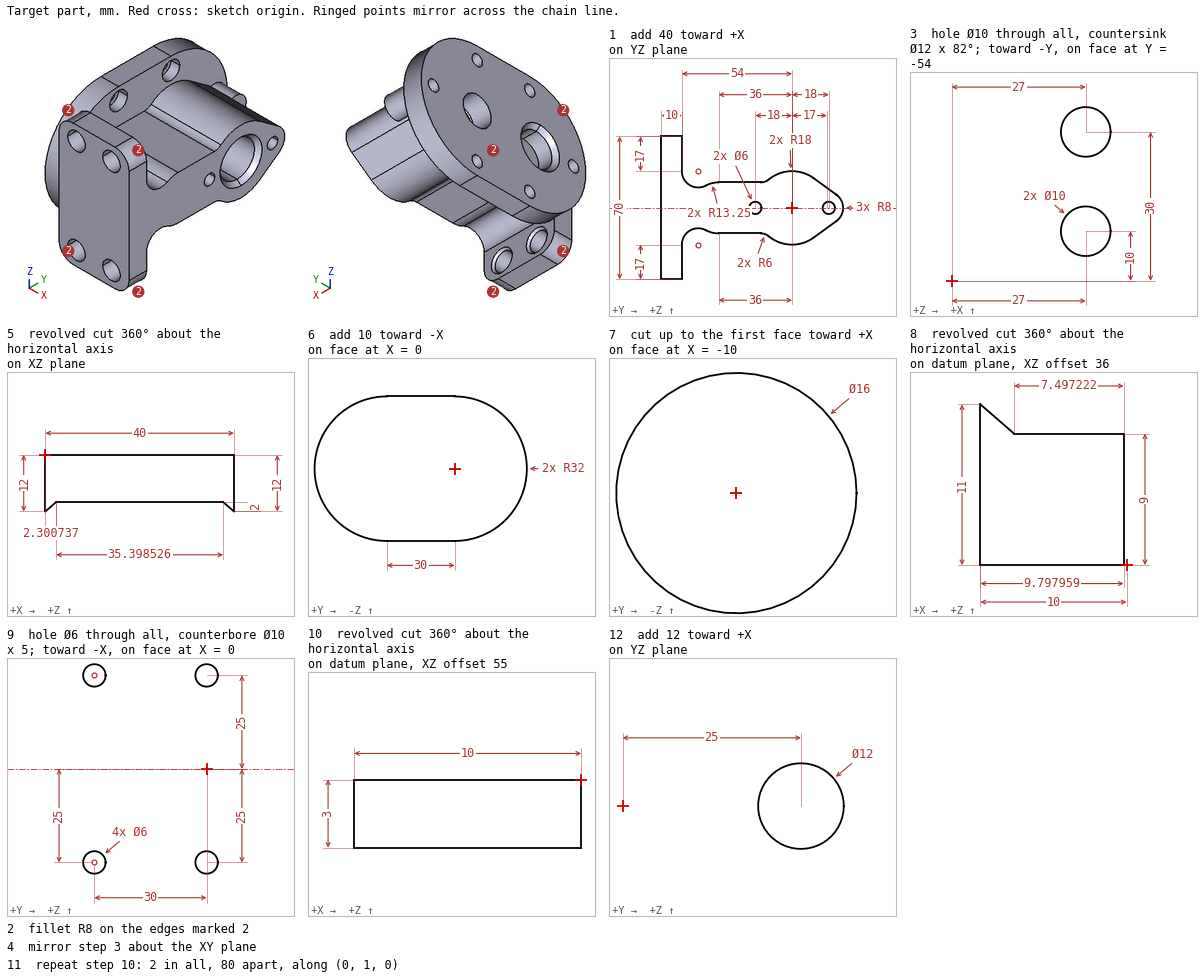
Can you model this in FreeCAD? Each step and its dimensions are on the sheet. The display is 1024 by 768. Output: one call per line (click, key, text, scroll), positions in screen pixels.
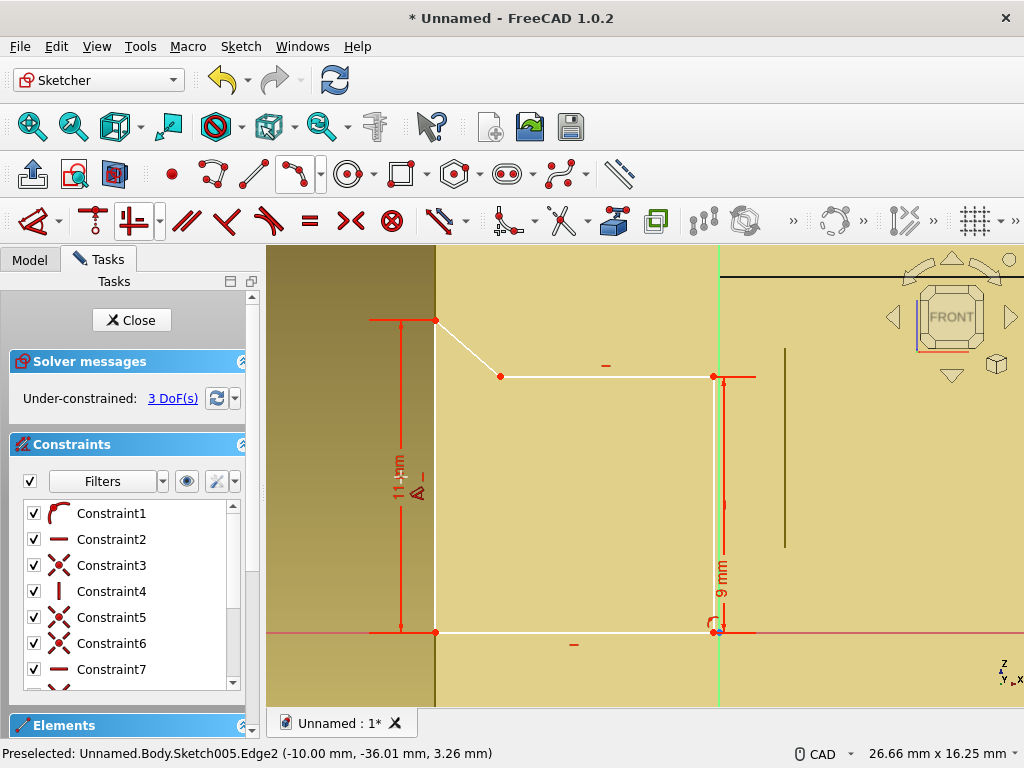
click(435, 633)
click(577, 667)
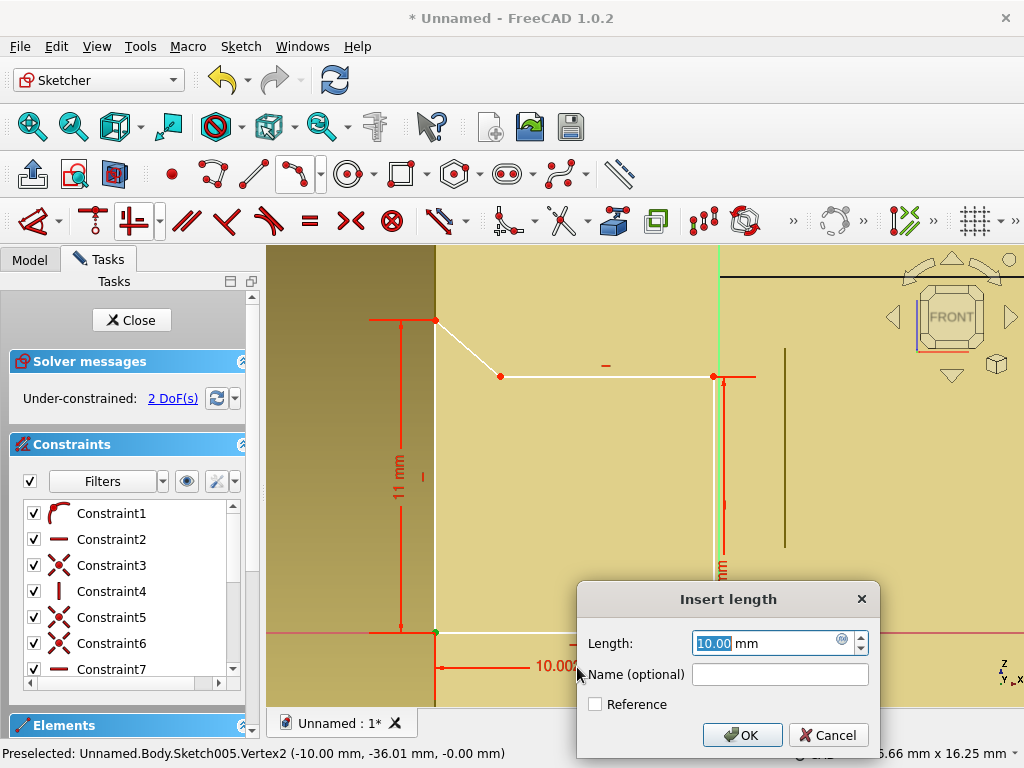
text(10)
key(Return)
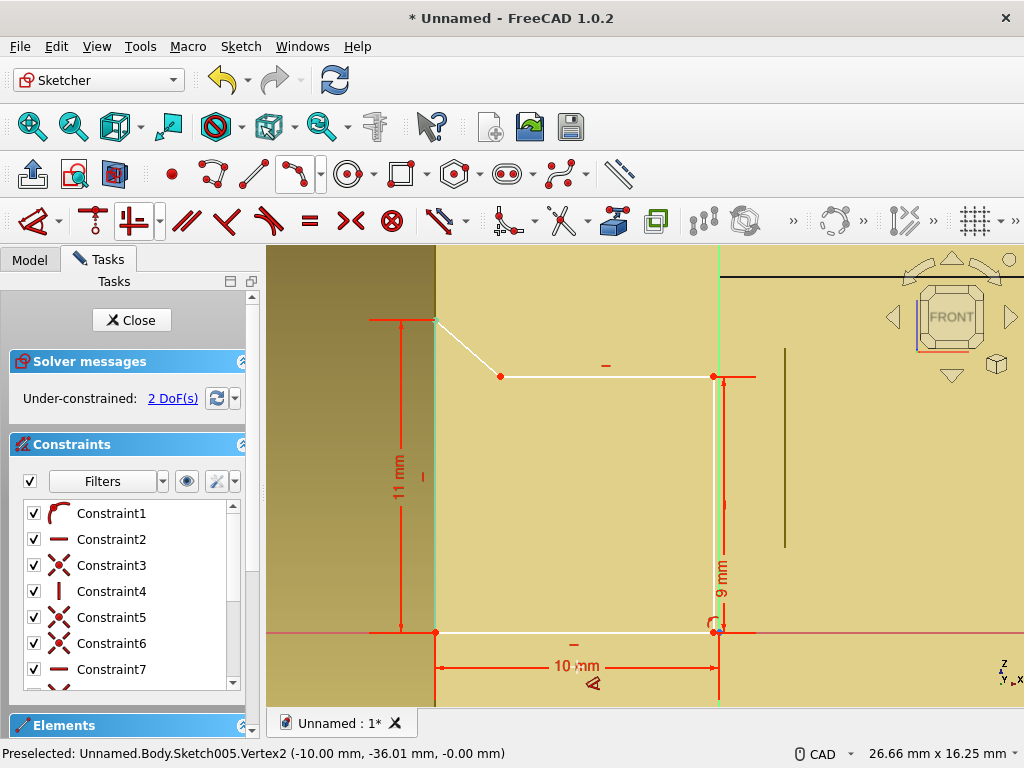
click(630, 633)
click(477, 667)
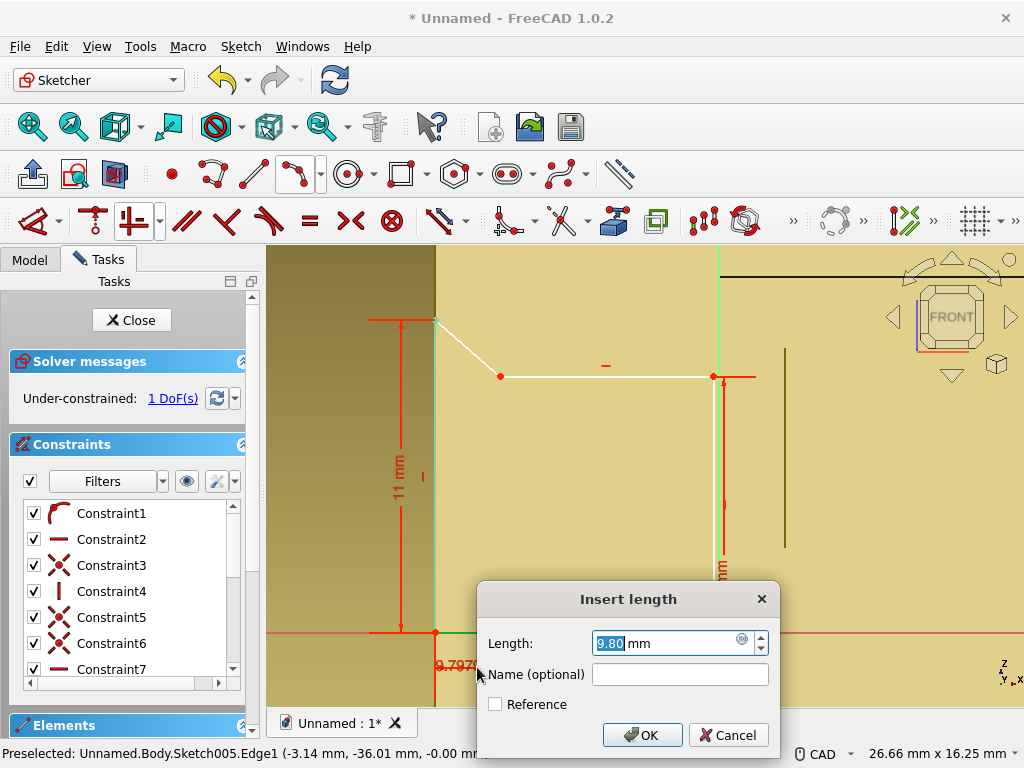
text(9.797959)
key(Return)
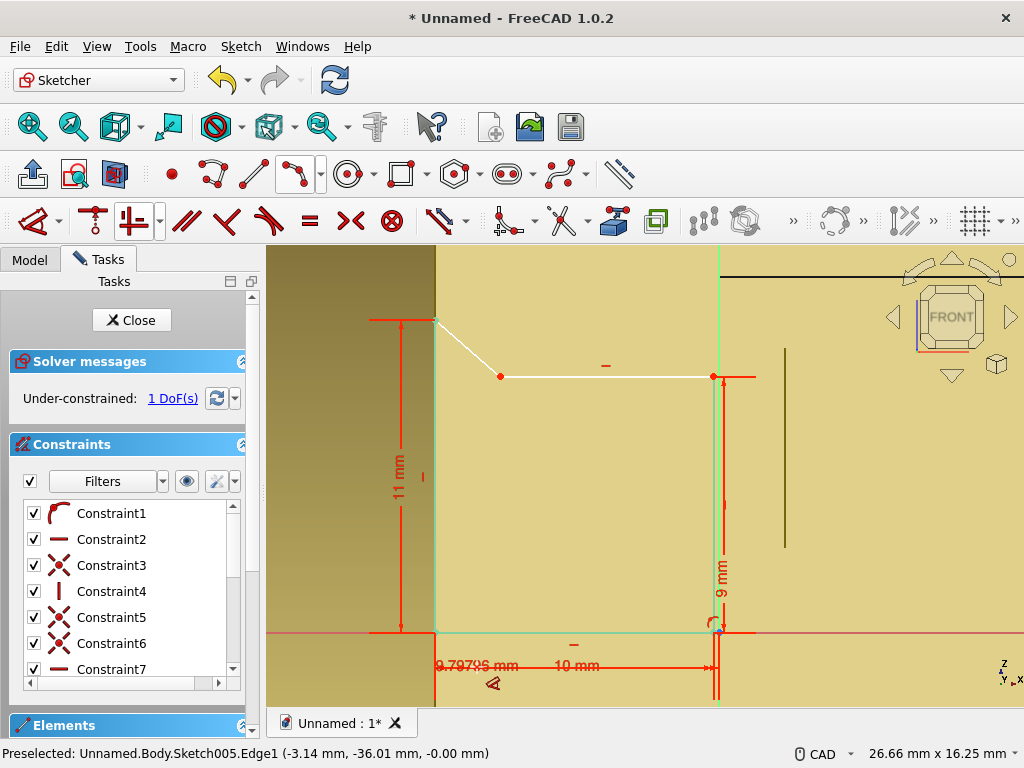
click(564, 377)
click(607, 343)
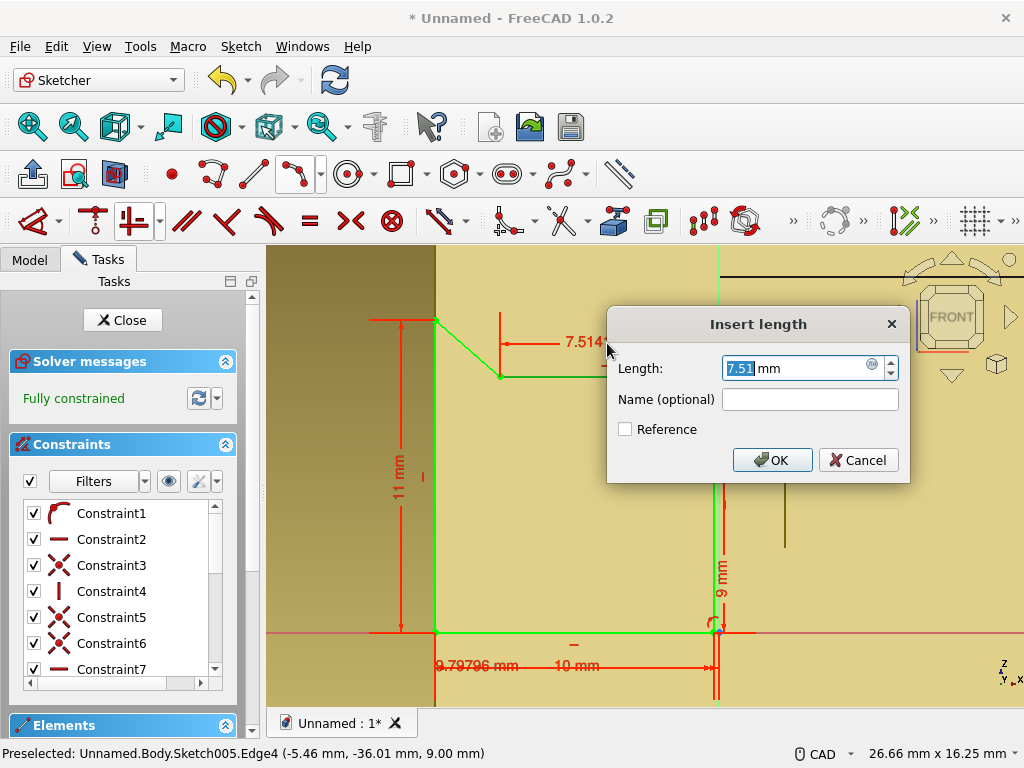
text(7.497222)
key(Return)
key(Escape)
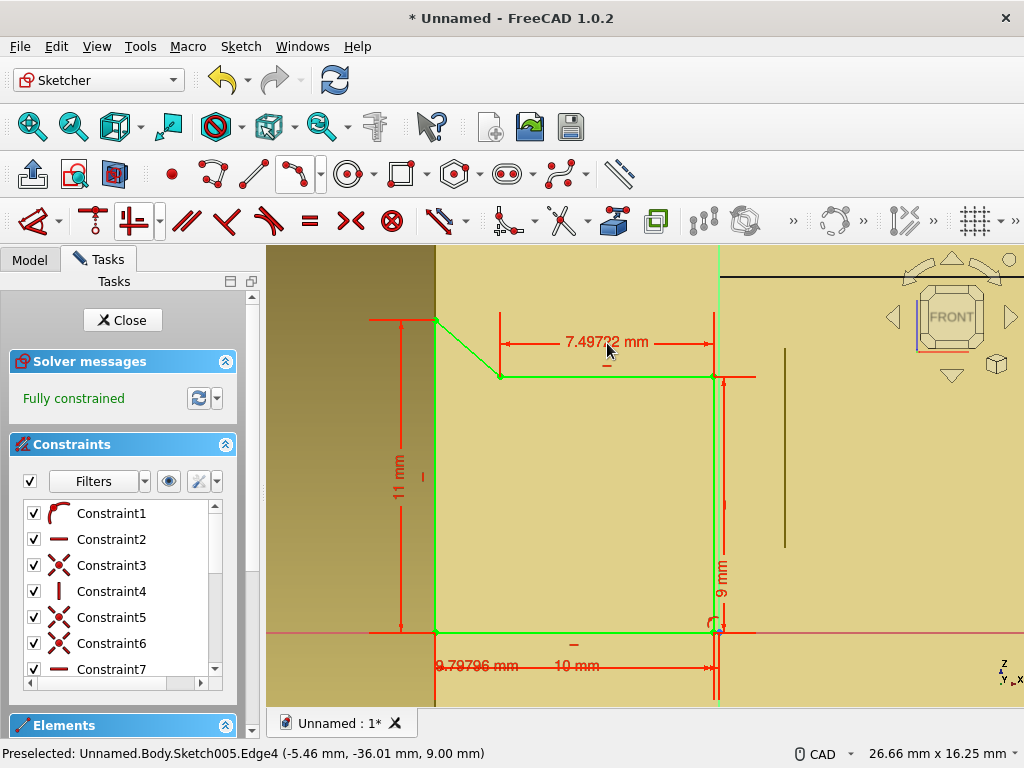
click(123, 320)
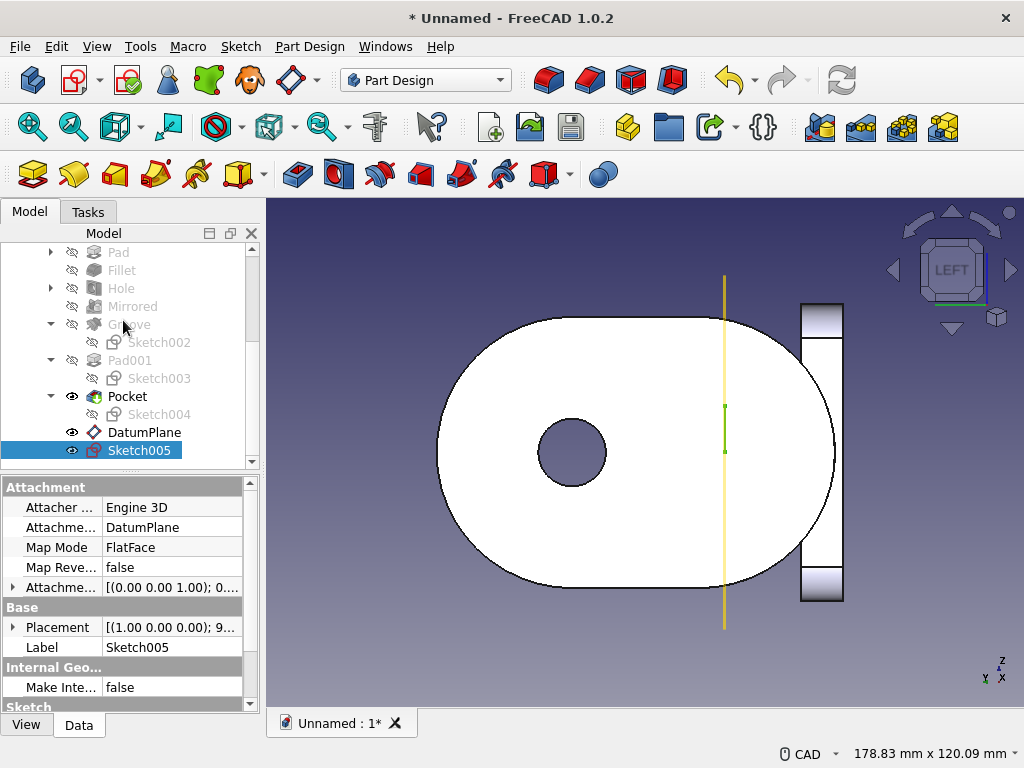
click(380, 174)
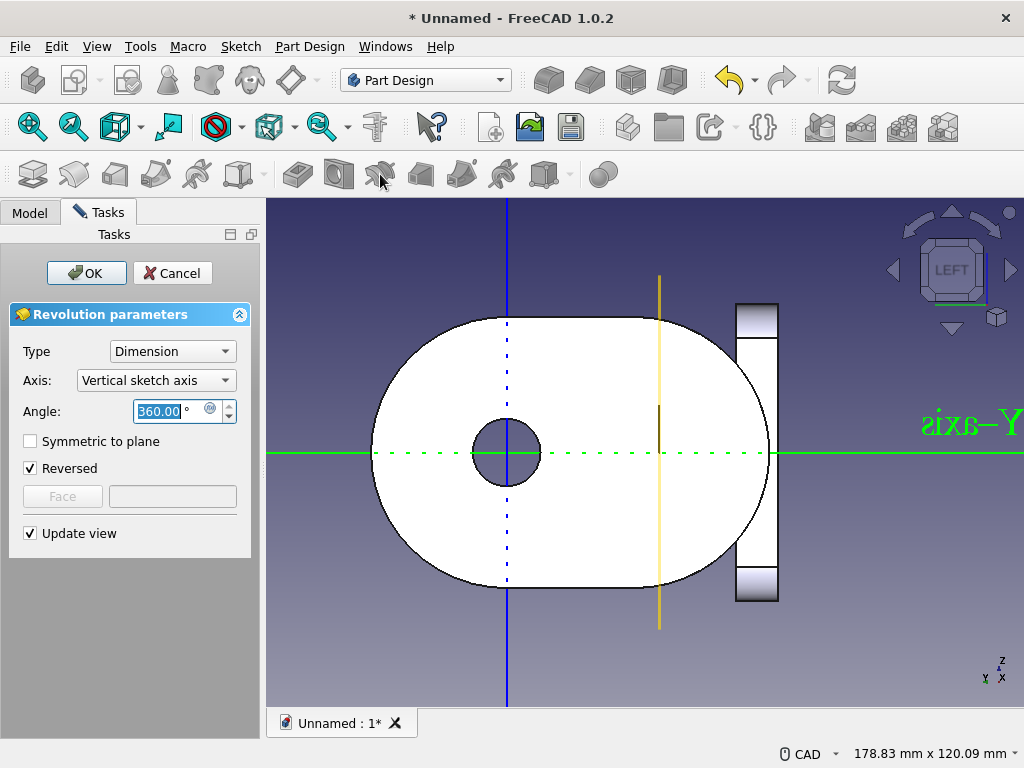
click(157, 380)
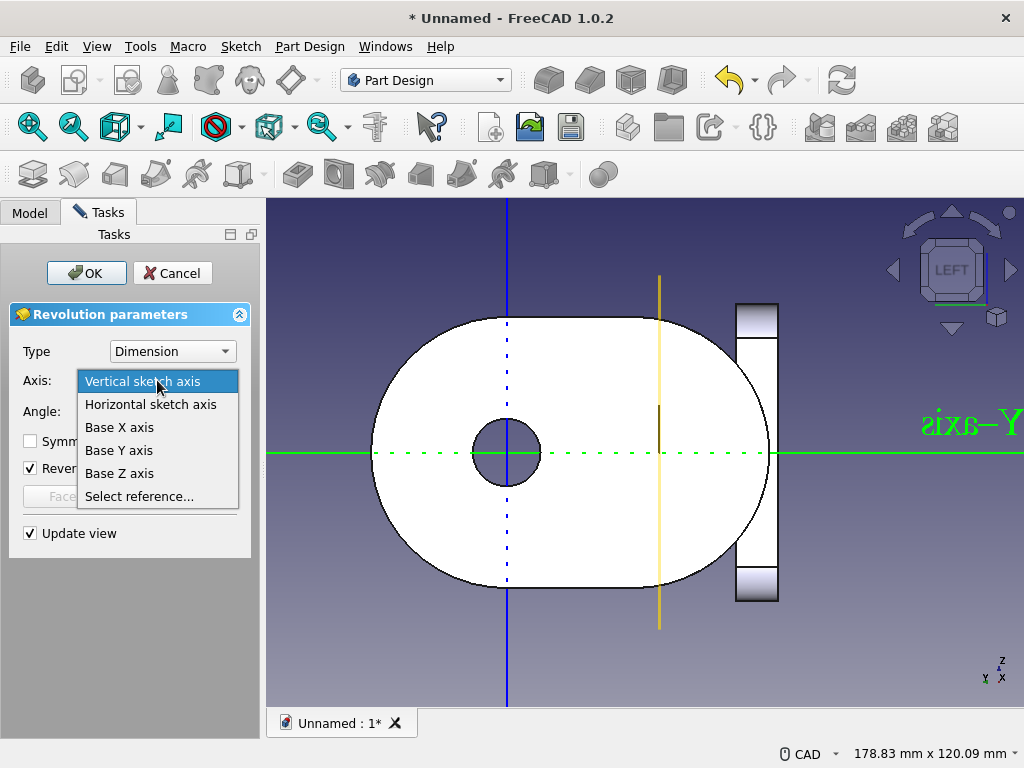
click(156, 404)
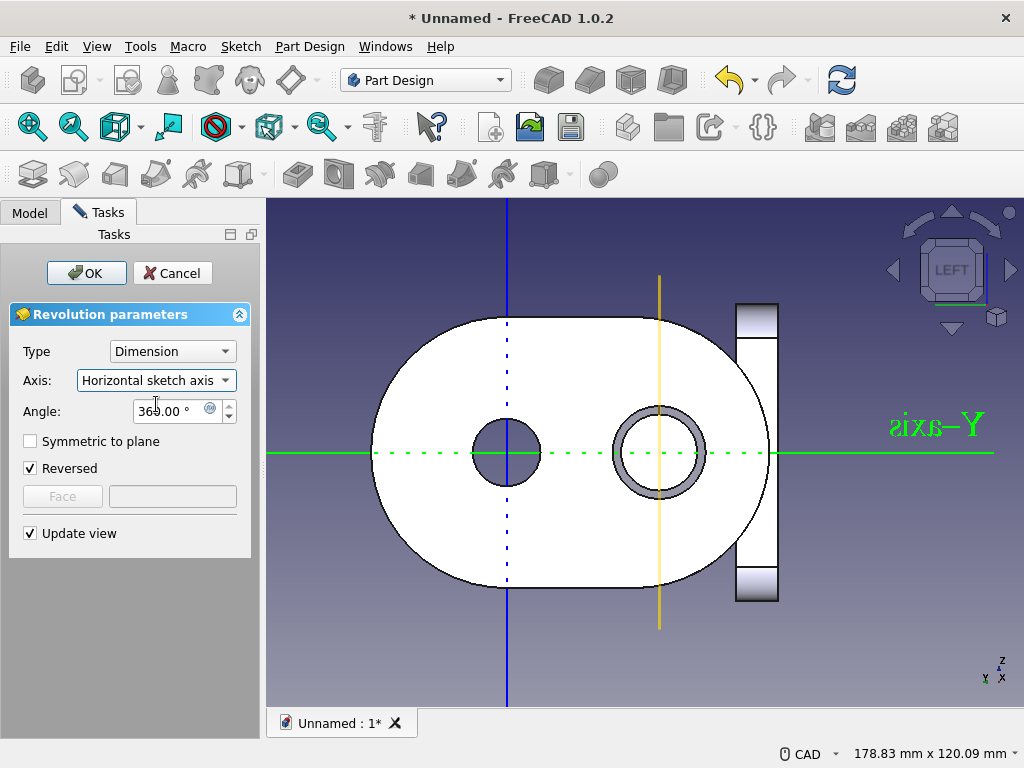
click(87, 273)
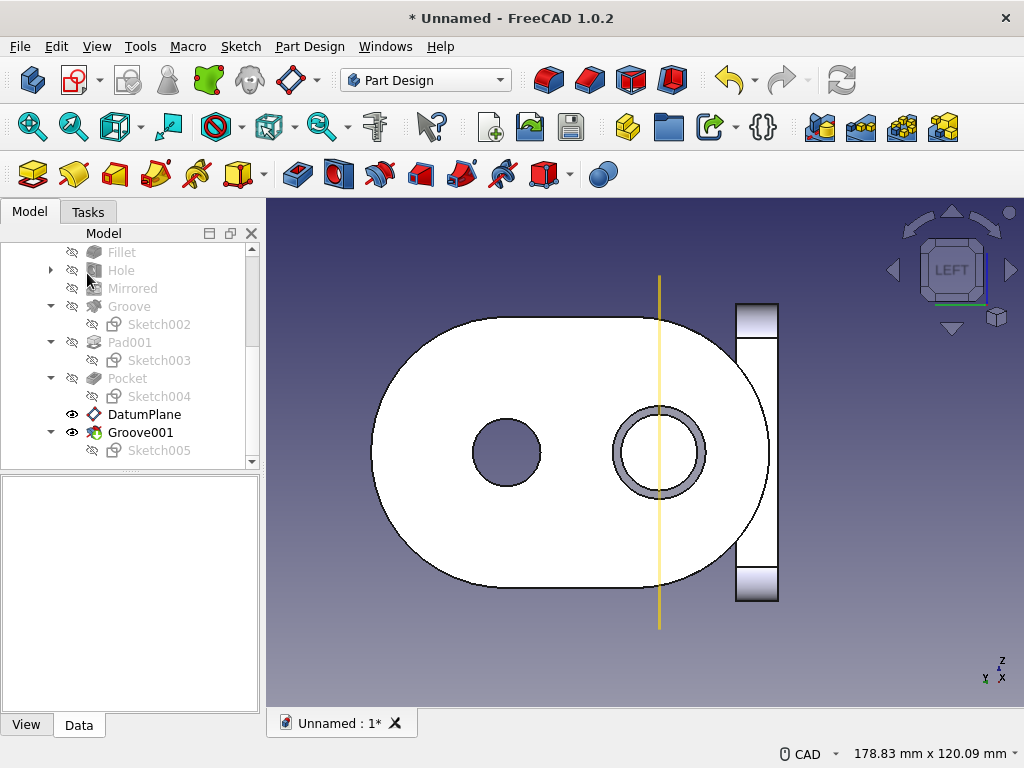
click(117, 414)
key(space)